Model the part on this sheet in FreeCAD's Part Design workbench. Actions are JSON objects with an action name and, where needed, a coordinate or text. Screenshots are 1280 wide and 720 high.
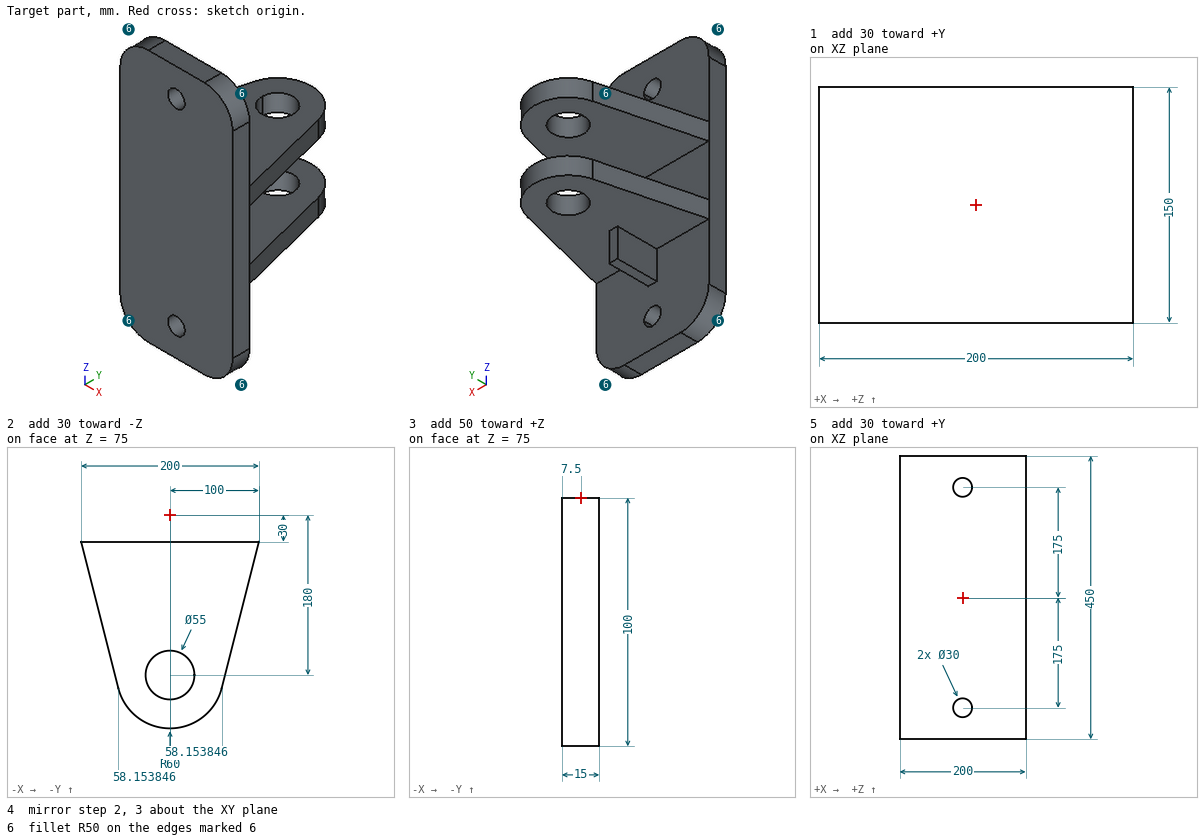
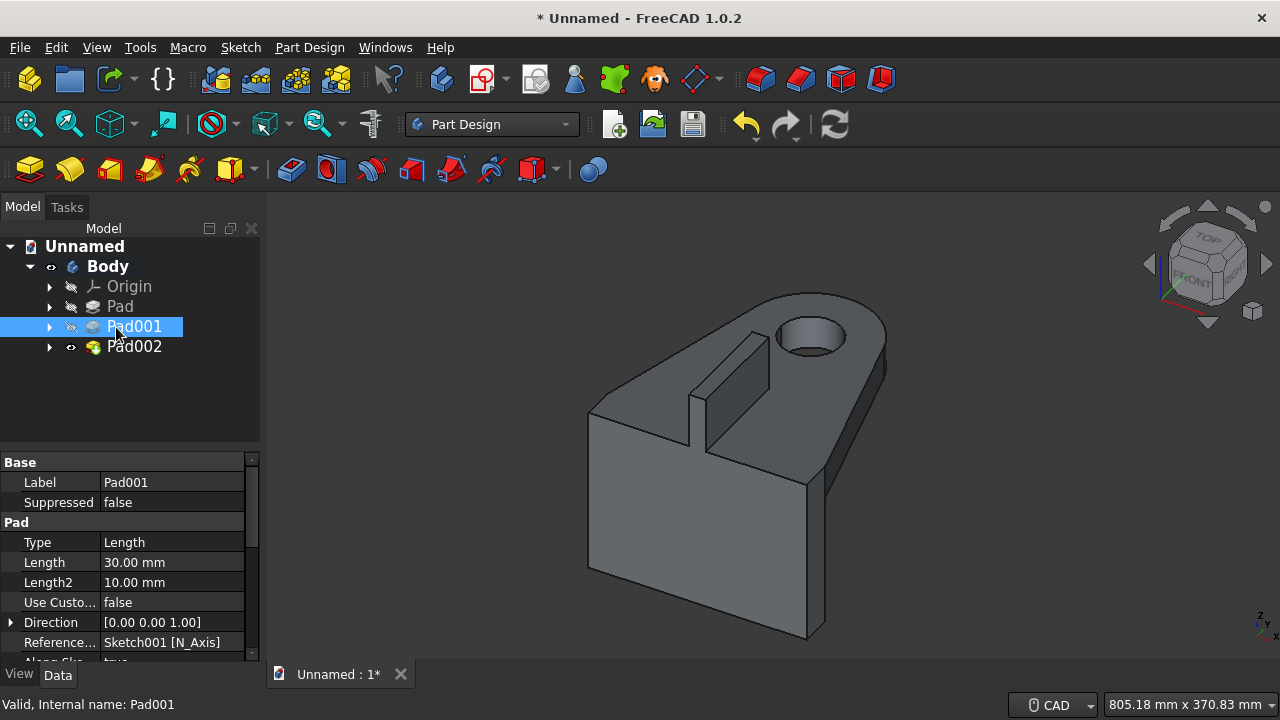
{"action": "left_click", "coordinate": [116, 347], "text": "ctrl"}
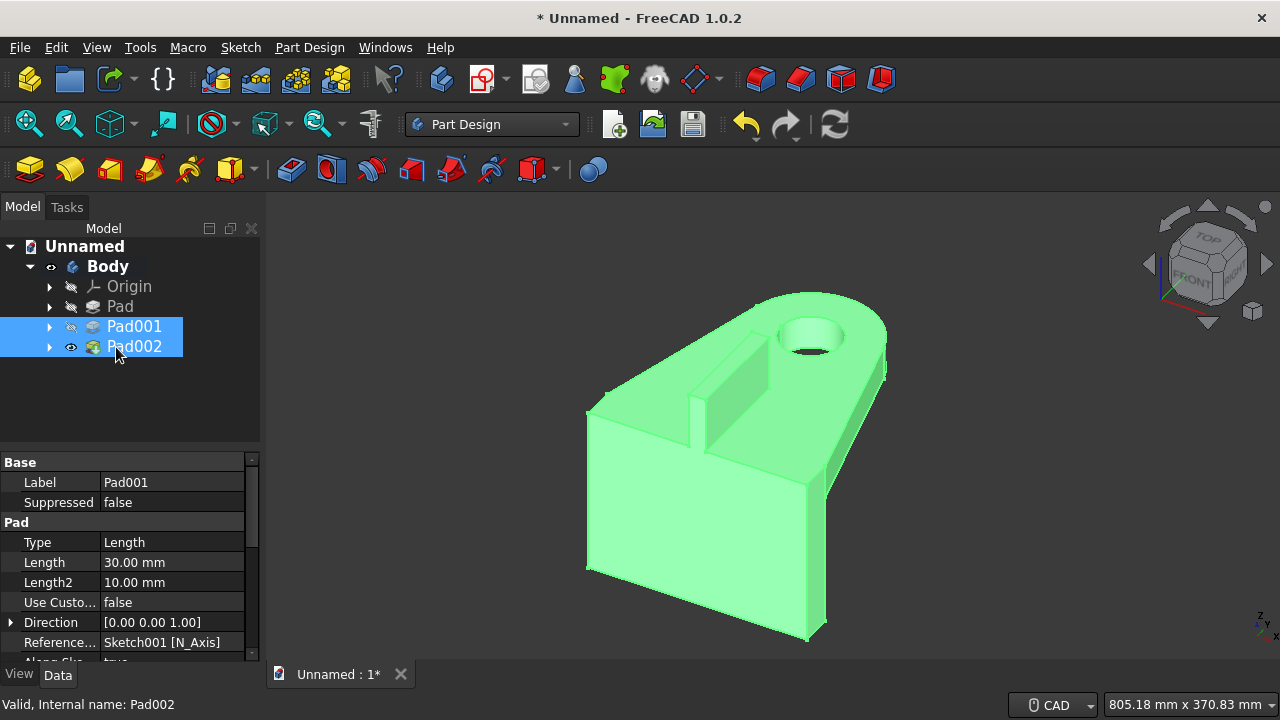
{"action": "left_click", "coordinate": [216, 80]}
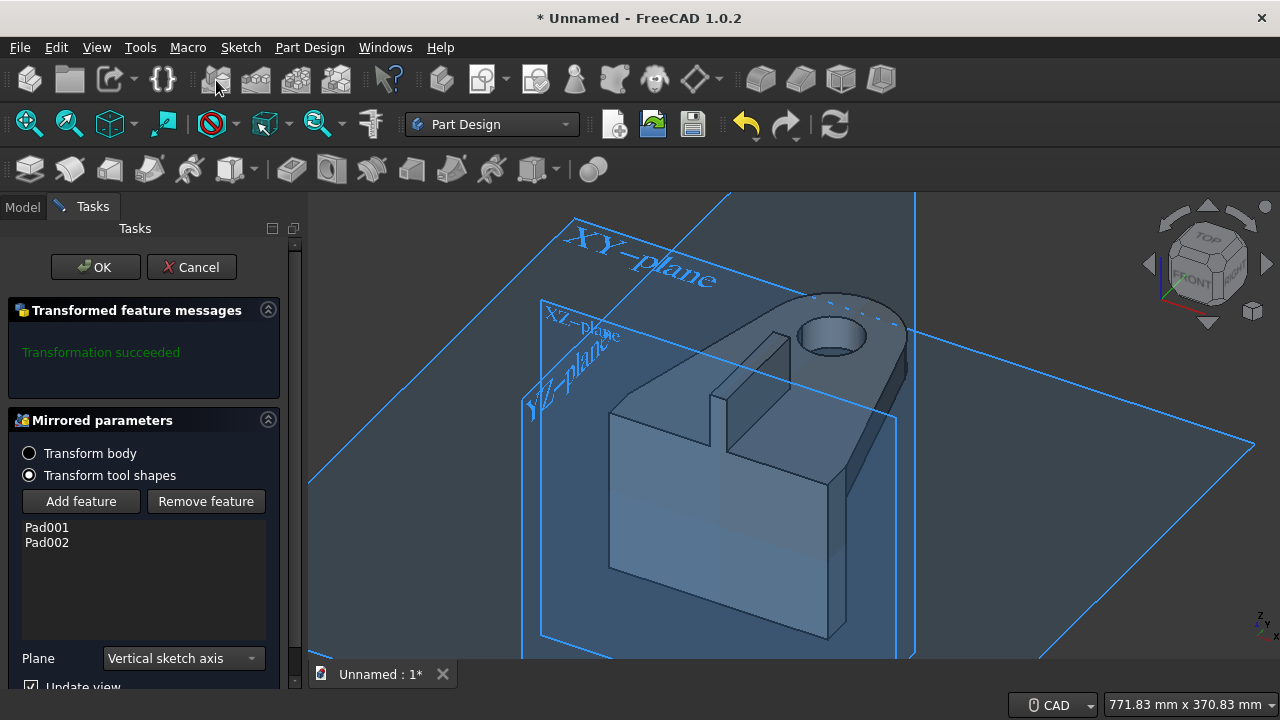
{"action": "left_click", "coordinate": [184, 658]}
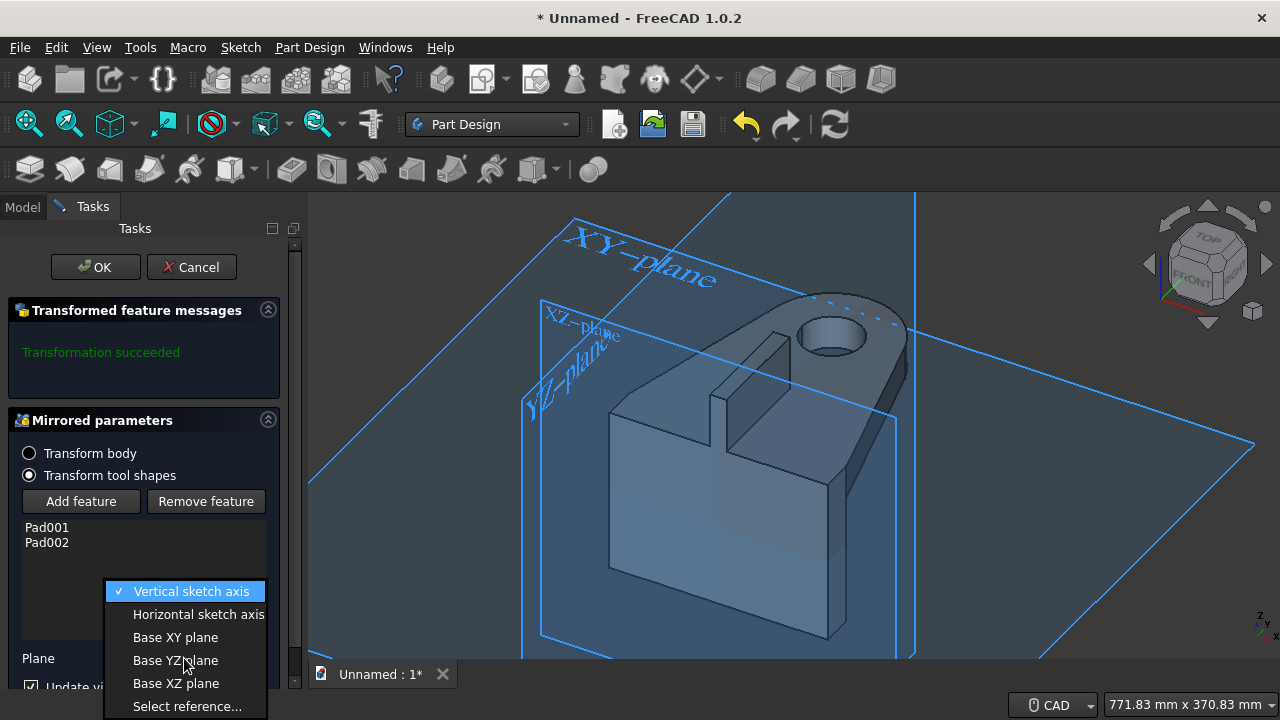
{"action": "left_click", "coordinate": [184, 638]}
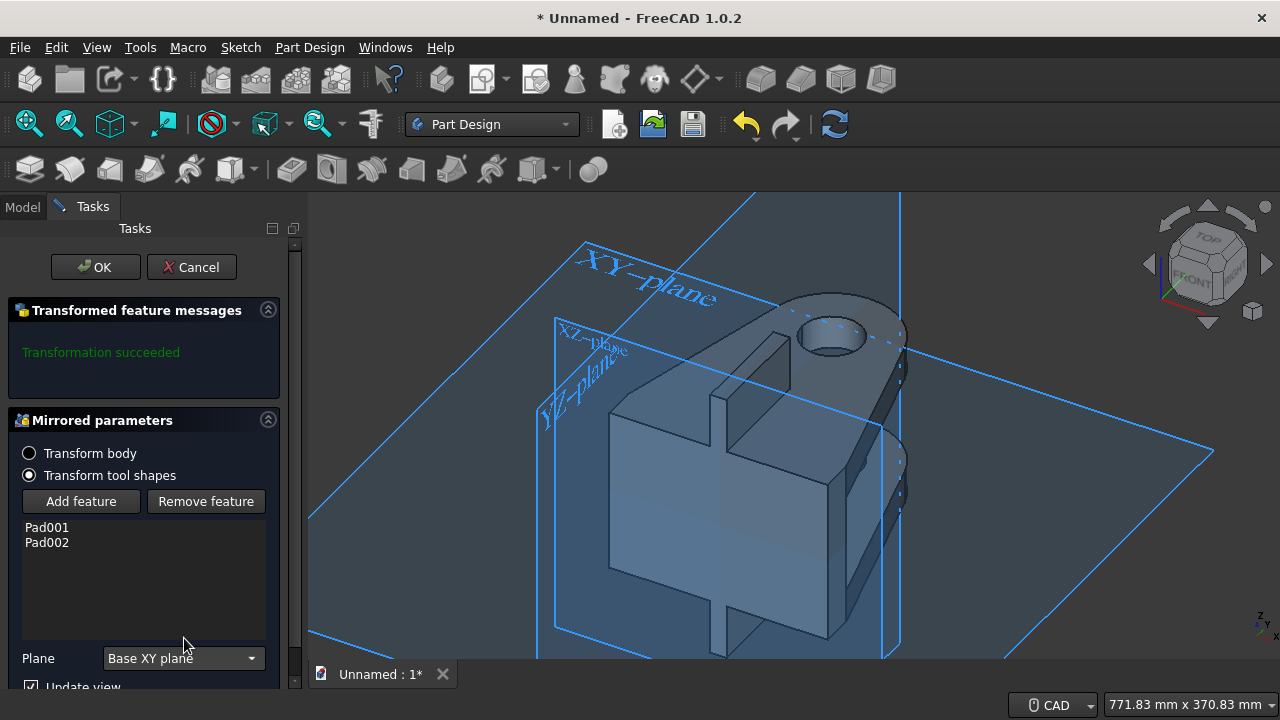
{"action": "left_click", "coordinate": [96, 267]}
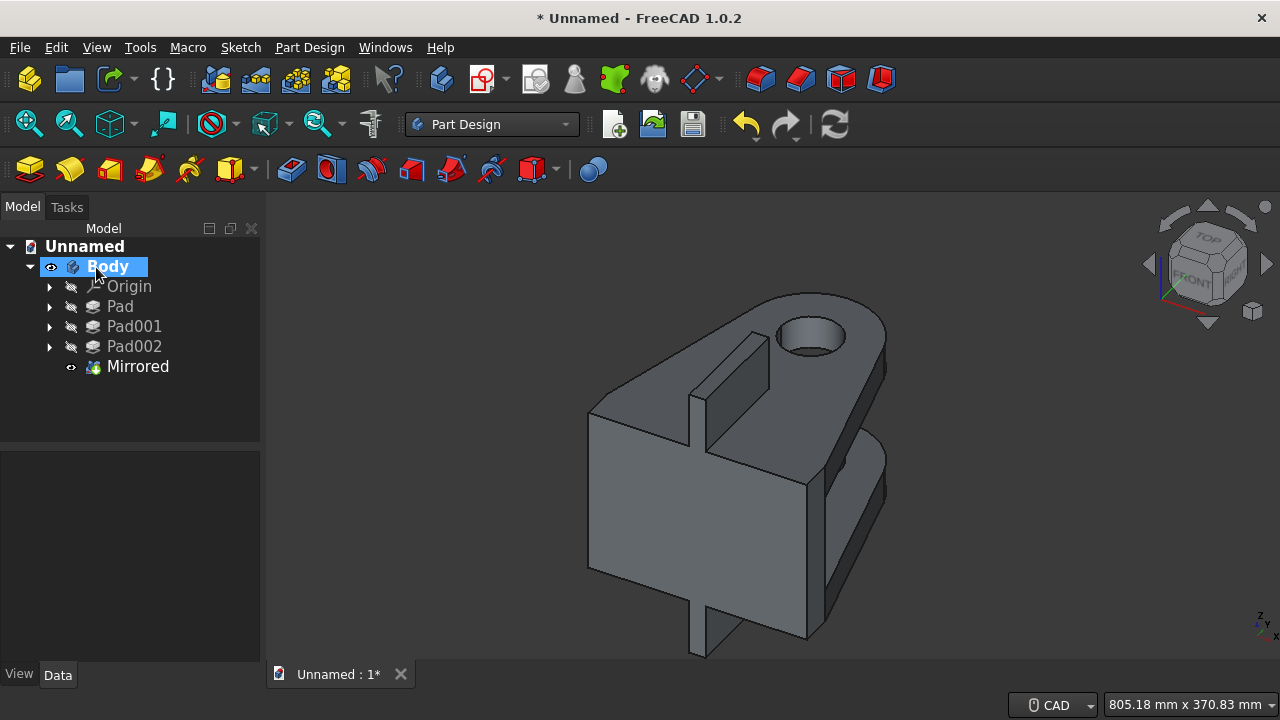
{"action": "left_click", "coordinate": [30, 124]}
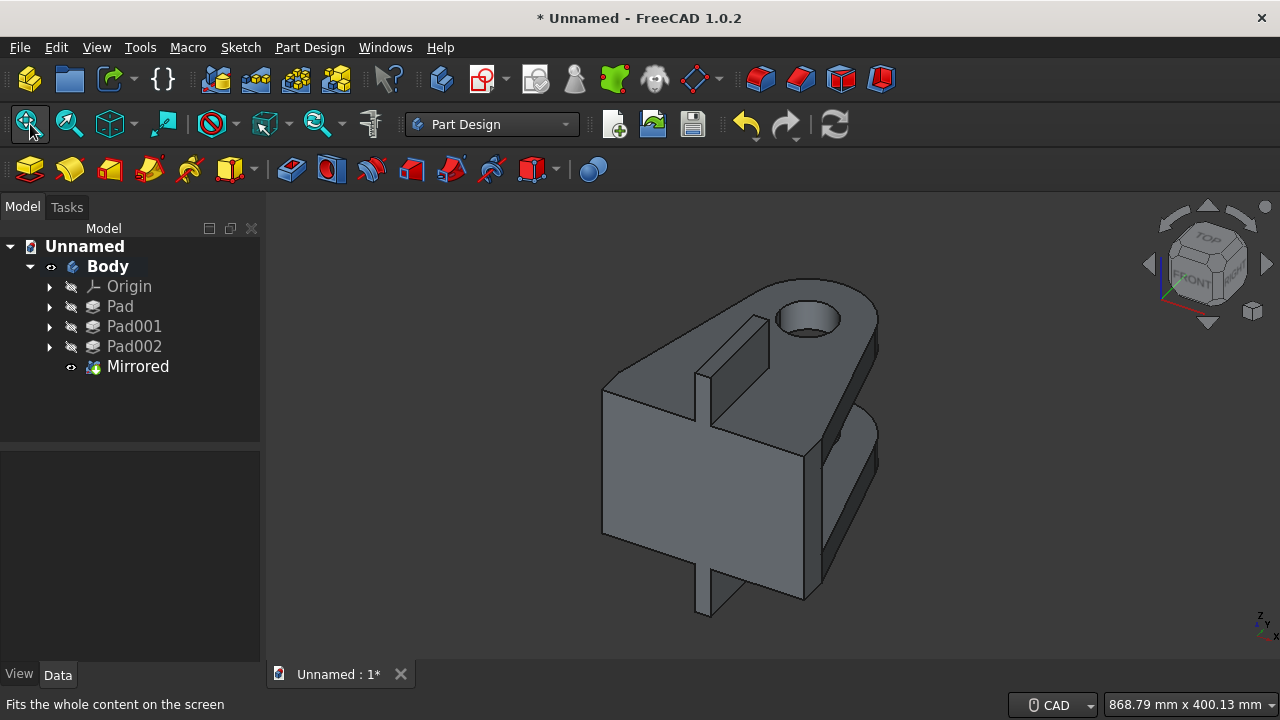
{"action": "left_click", "coordinate": [482, 80]}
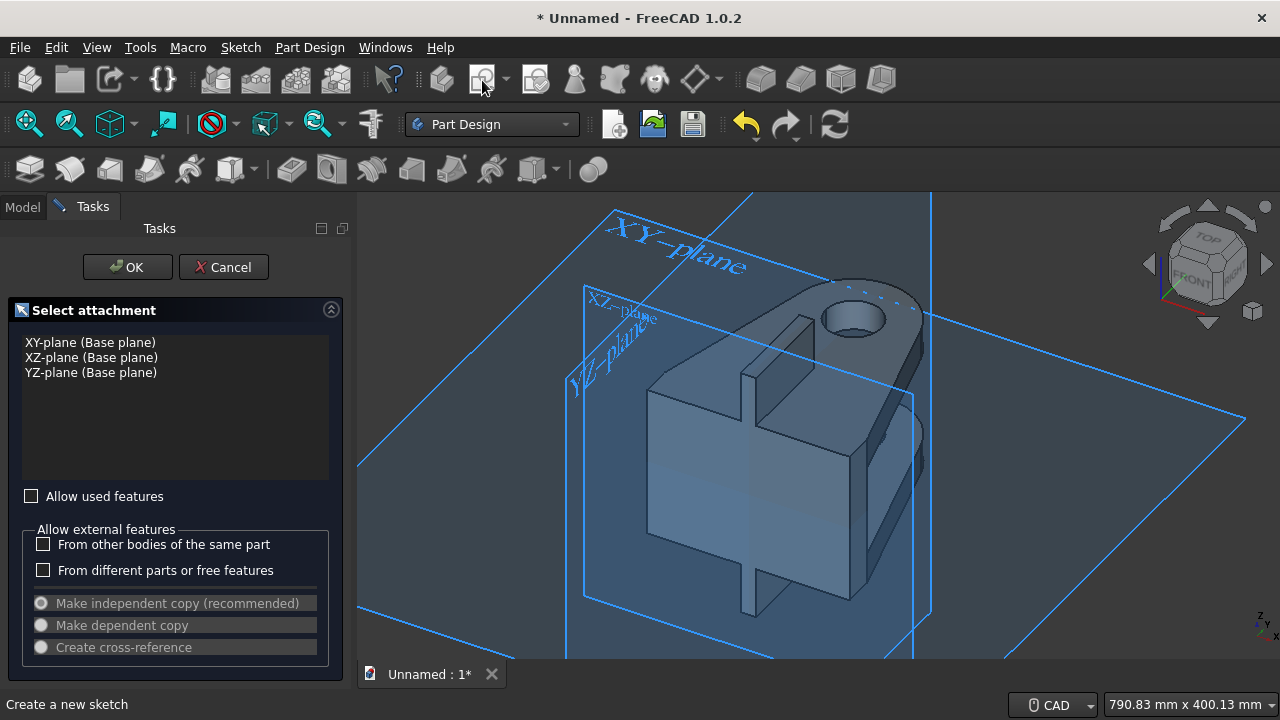
{"action": "left_click", "coordinate": [82, 358]}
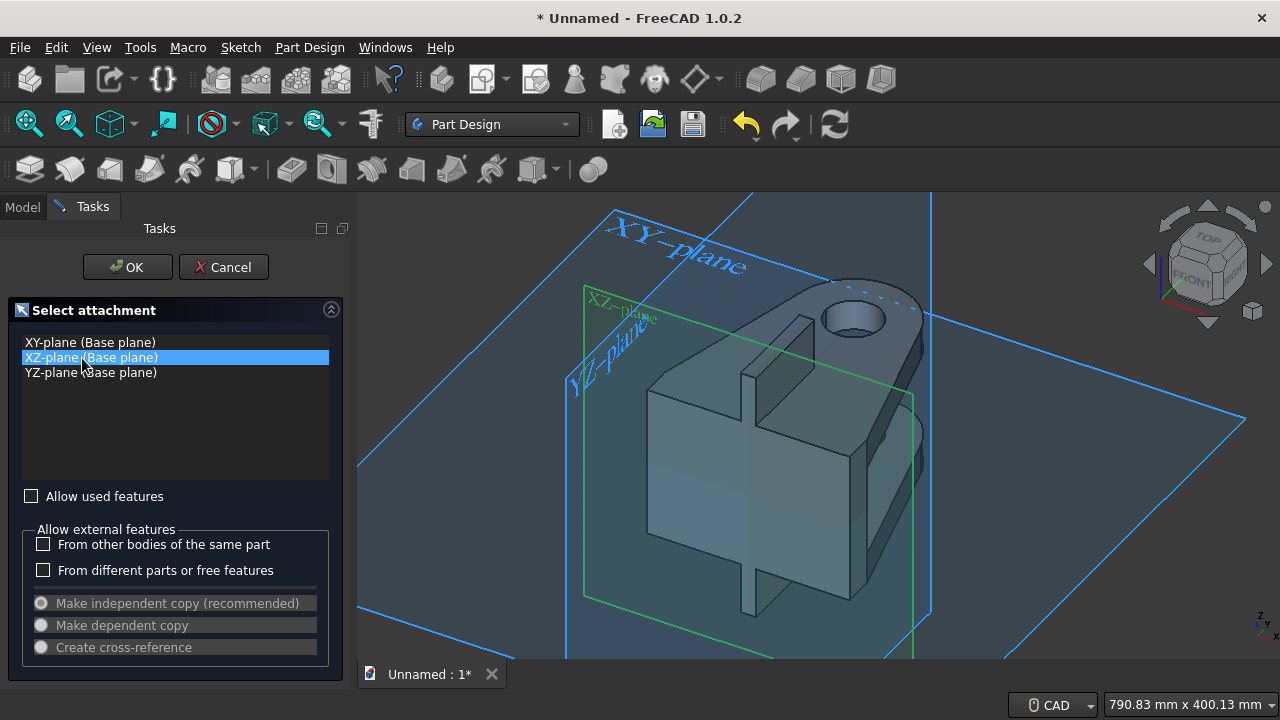
{"action": "left_click", "coordinate": [128, 267]}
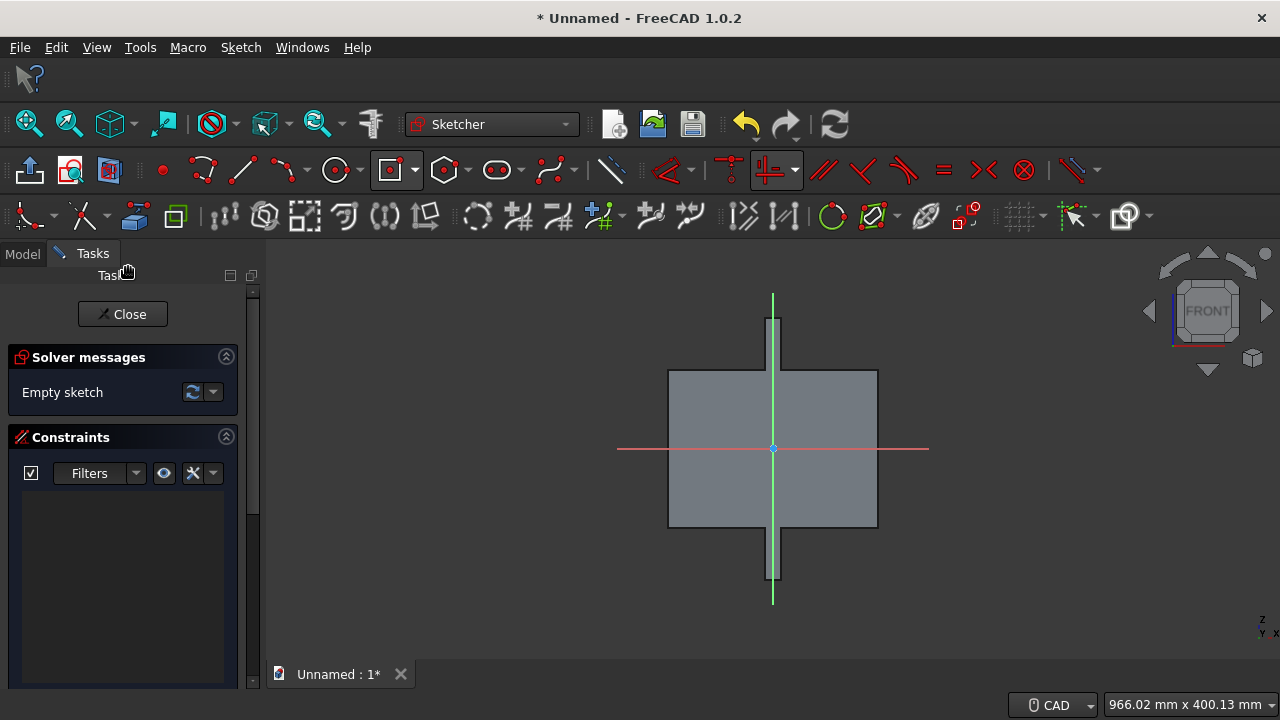
{"action": "scroll", "coordinate": [621, 449], "scroll_direction": "down", "scroll_amount": 3}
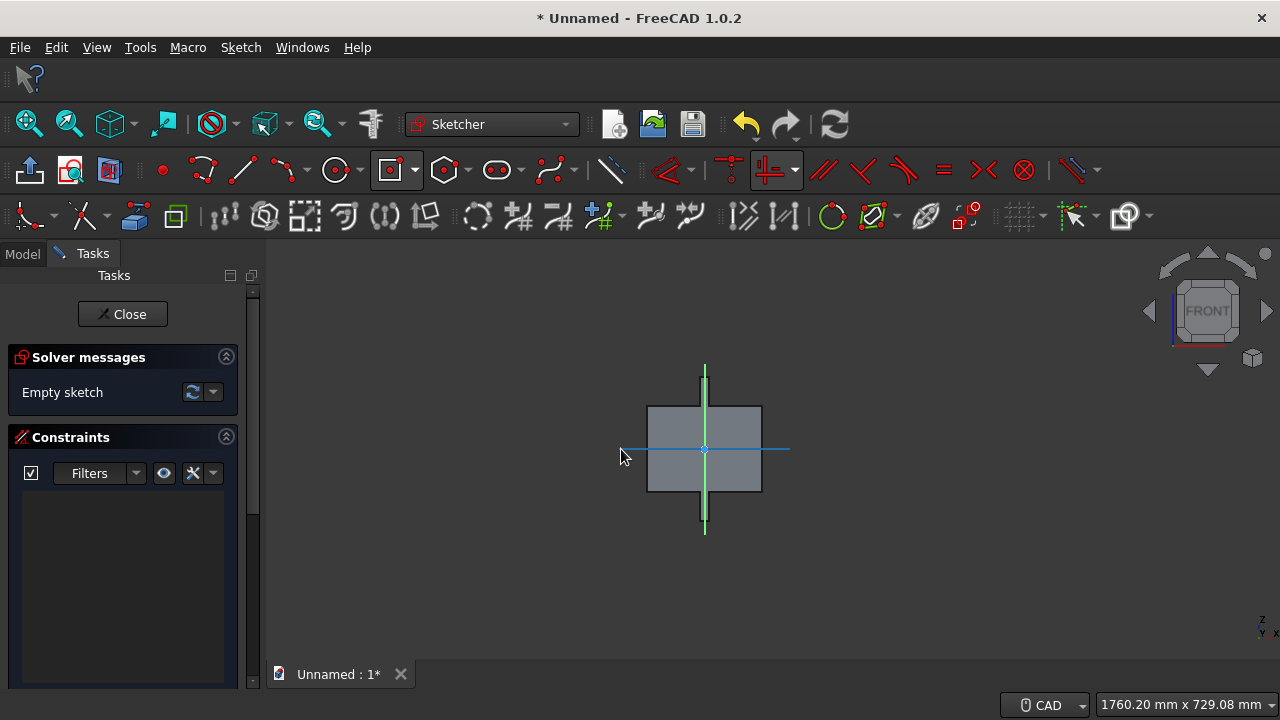
{"action": "key", "text": "g v"}